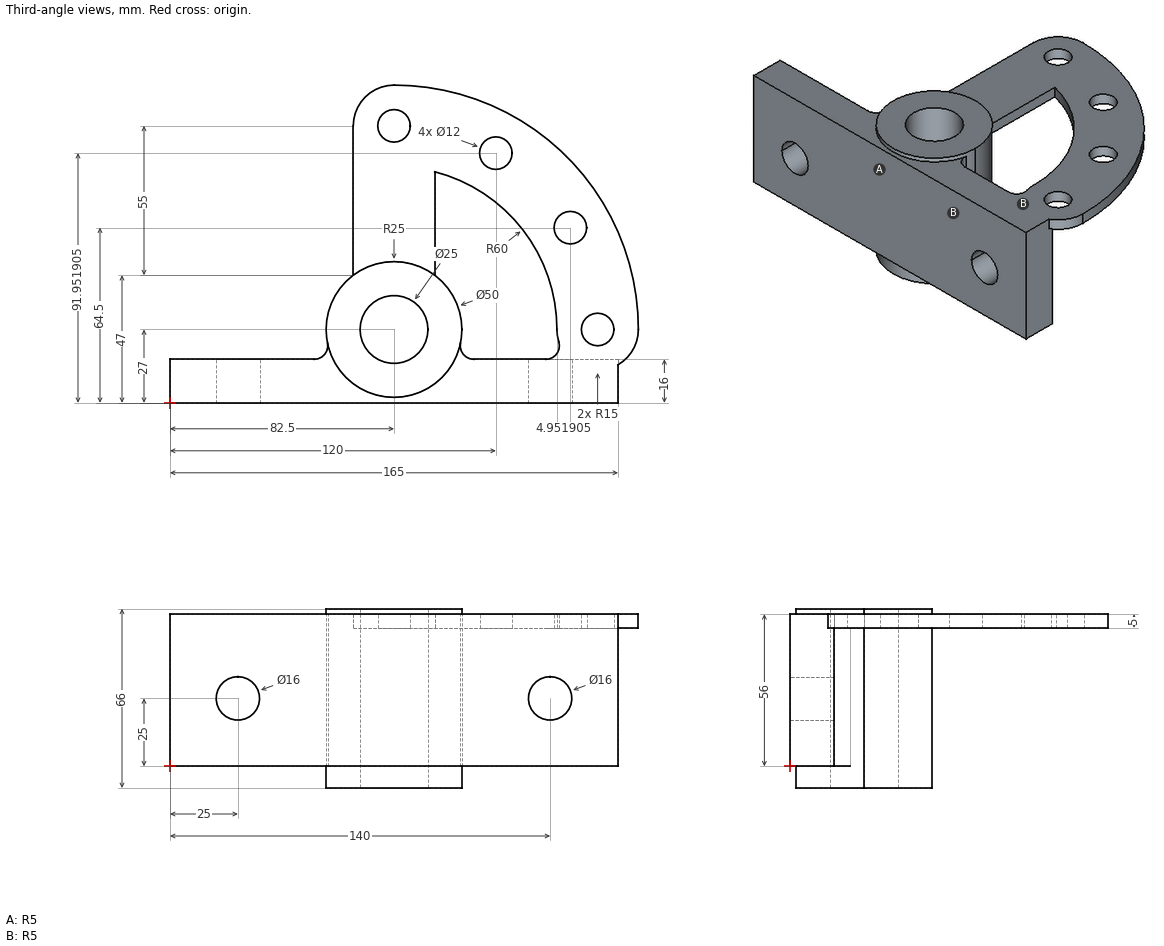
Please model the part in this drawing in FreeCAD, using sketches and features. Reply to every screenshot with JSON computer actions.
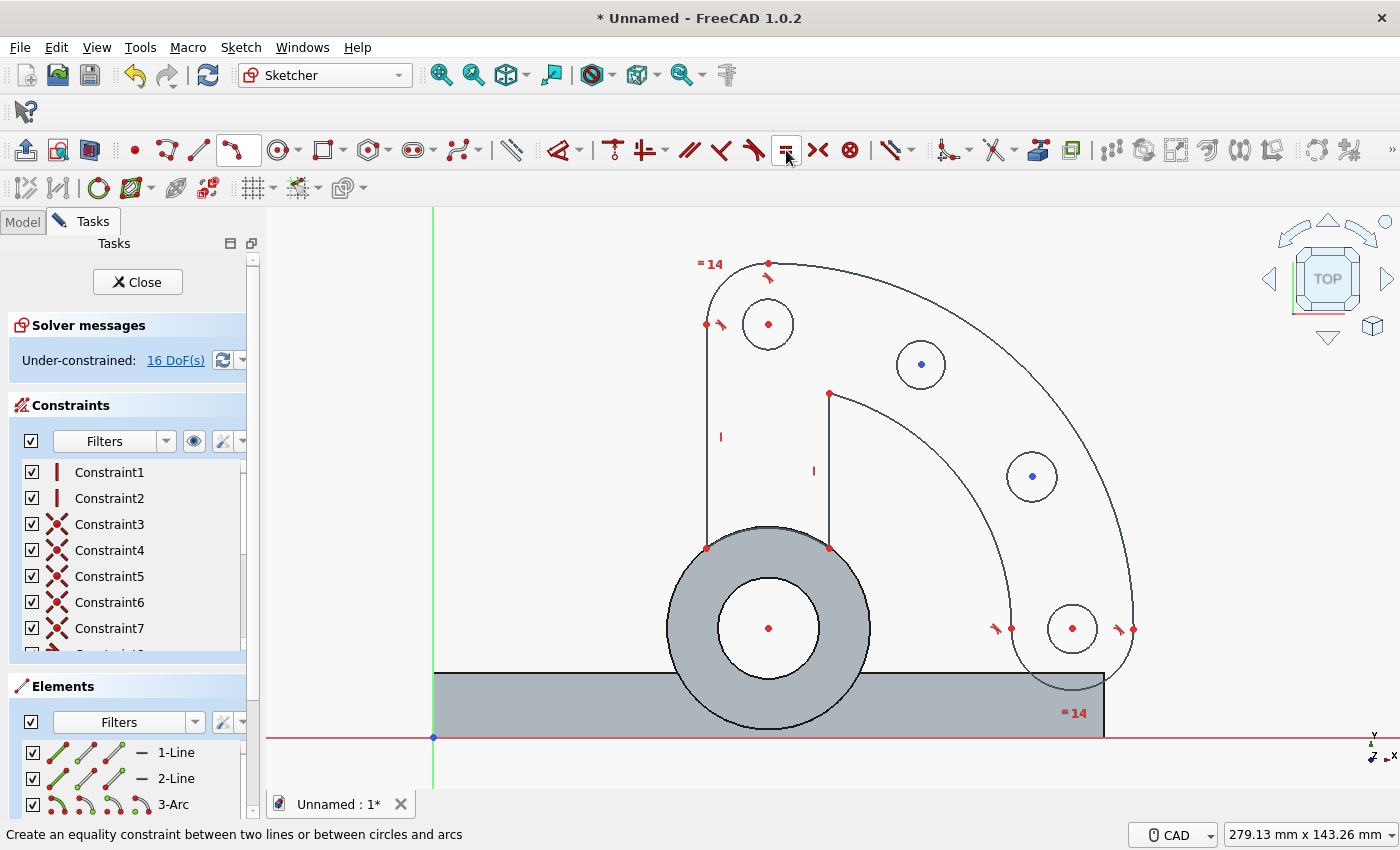
{"action": "left_click", "coordinate": [938, 348]}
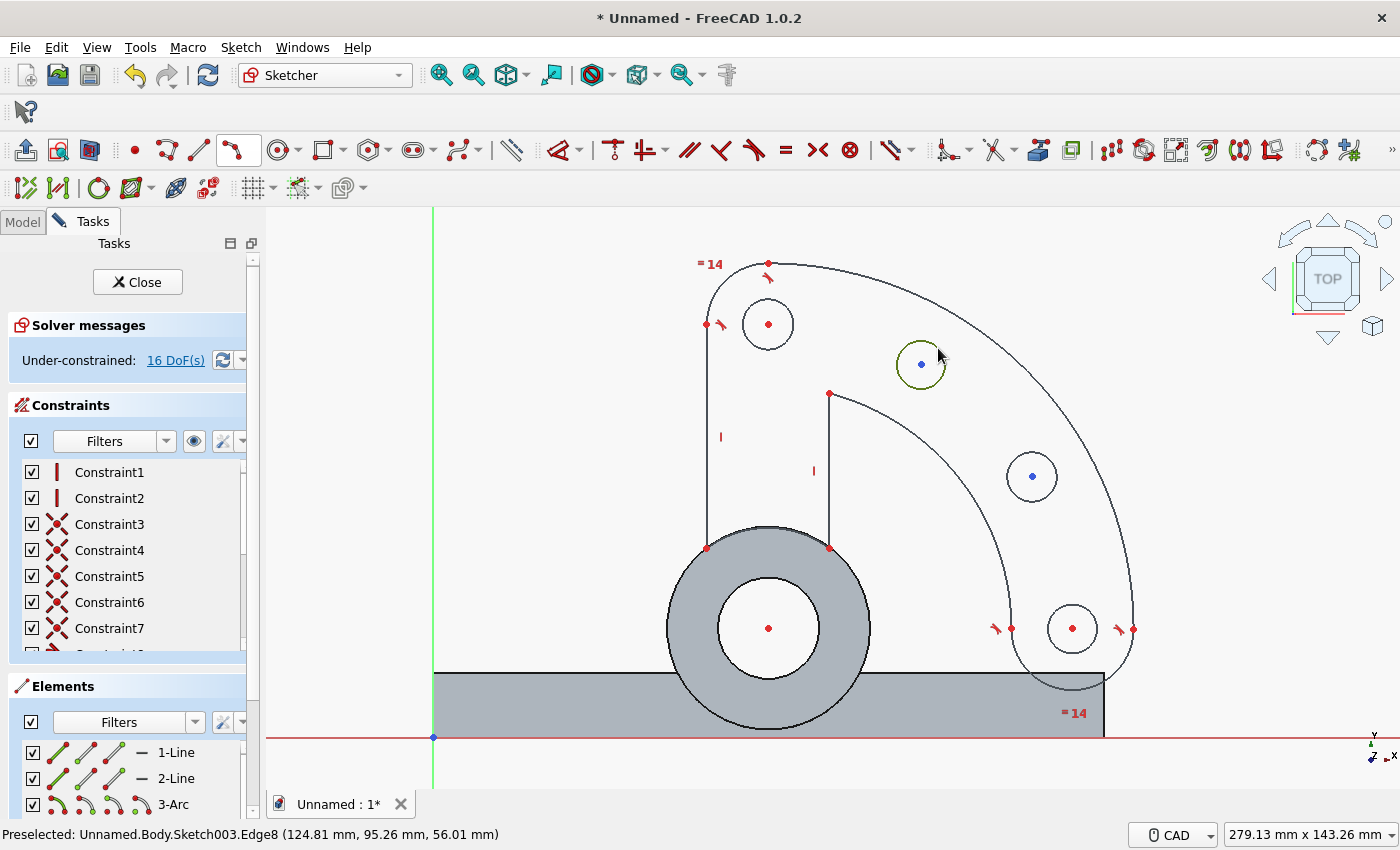
{"action": "left_click", "coordinate": [786, 307]}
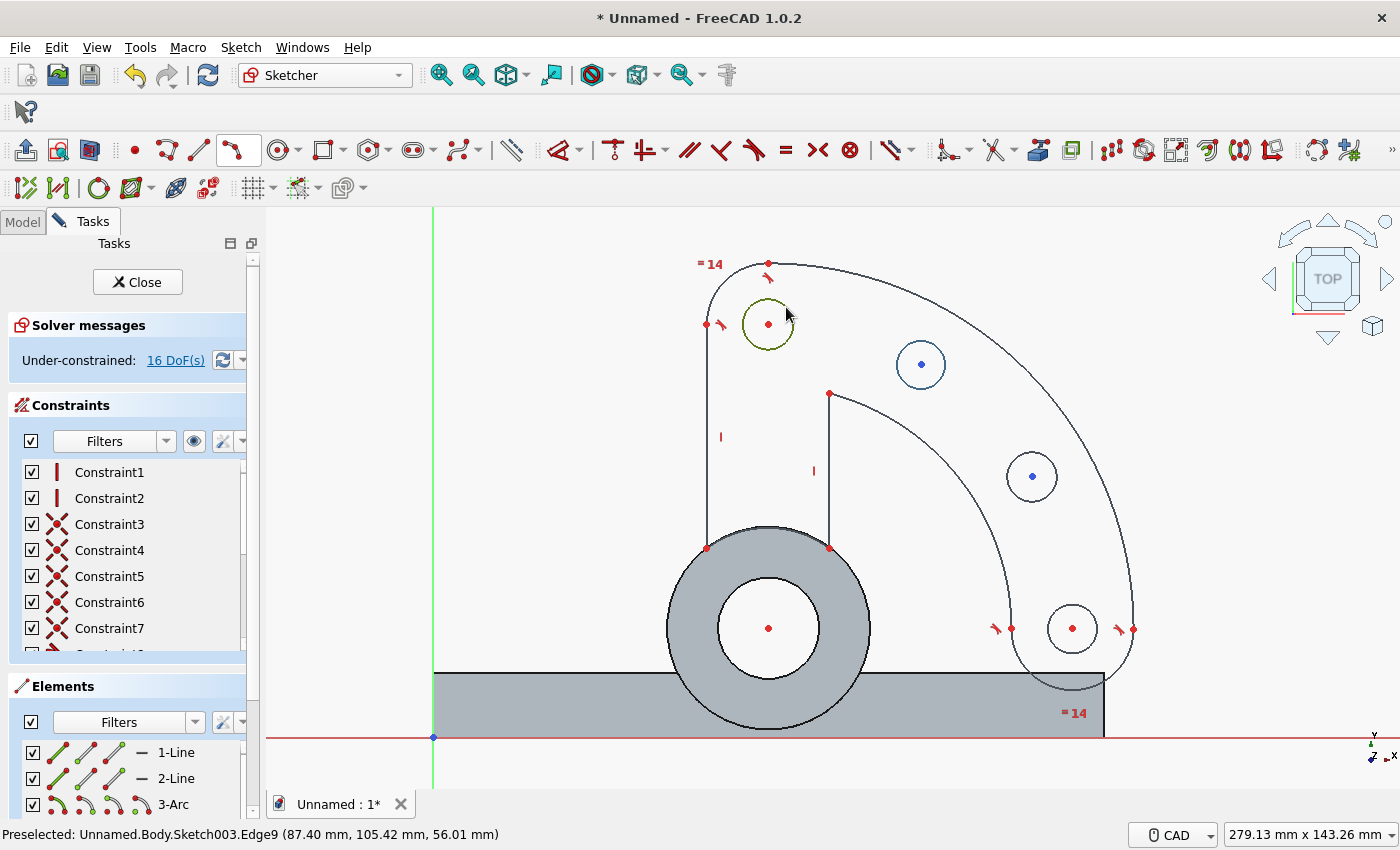
{"action": "left_click", "coordinate": [1090, 612]}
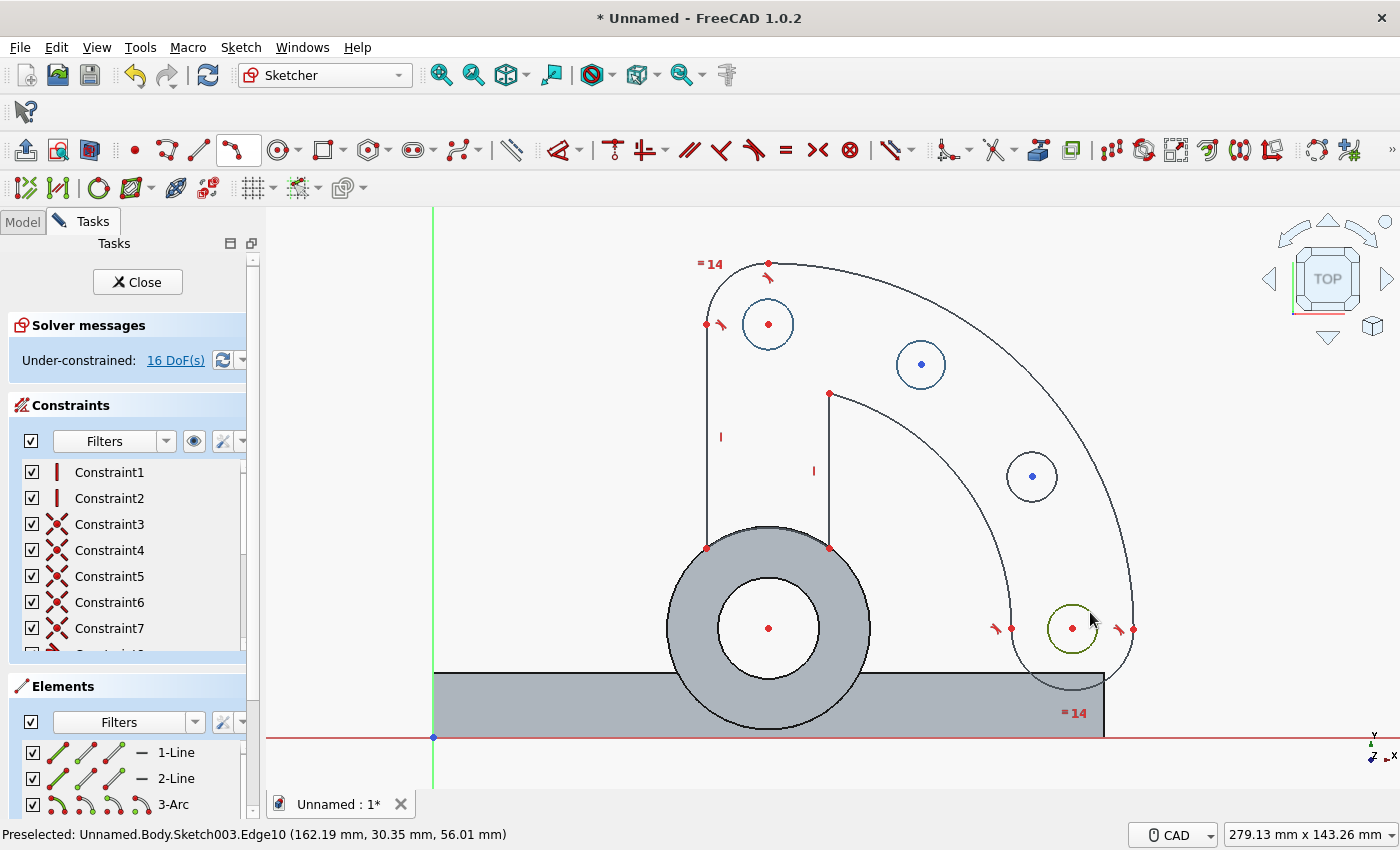
{"action": "left_click", "coordinate": [1049, 459]}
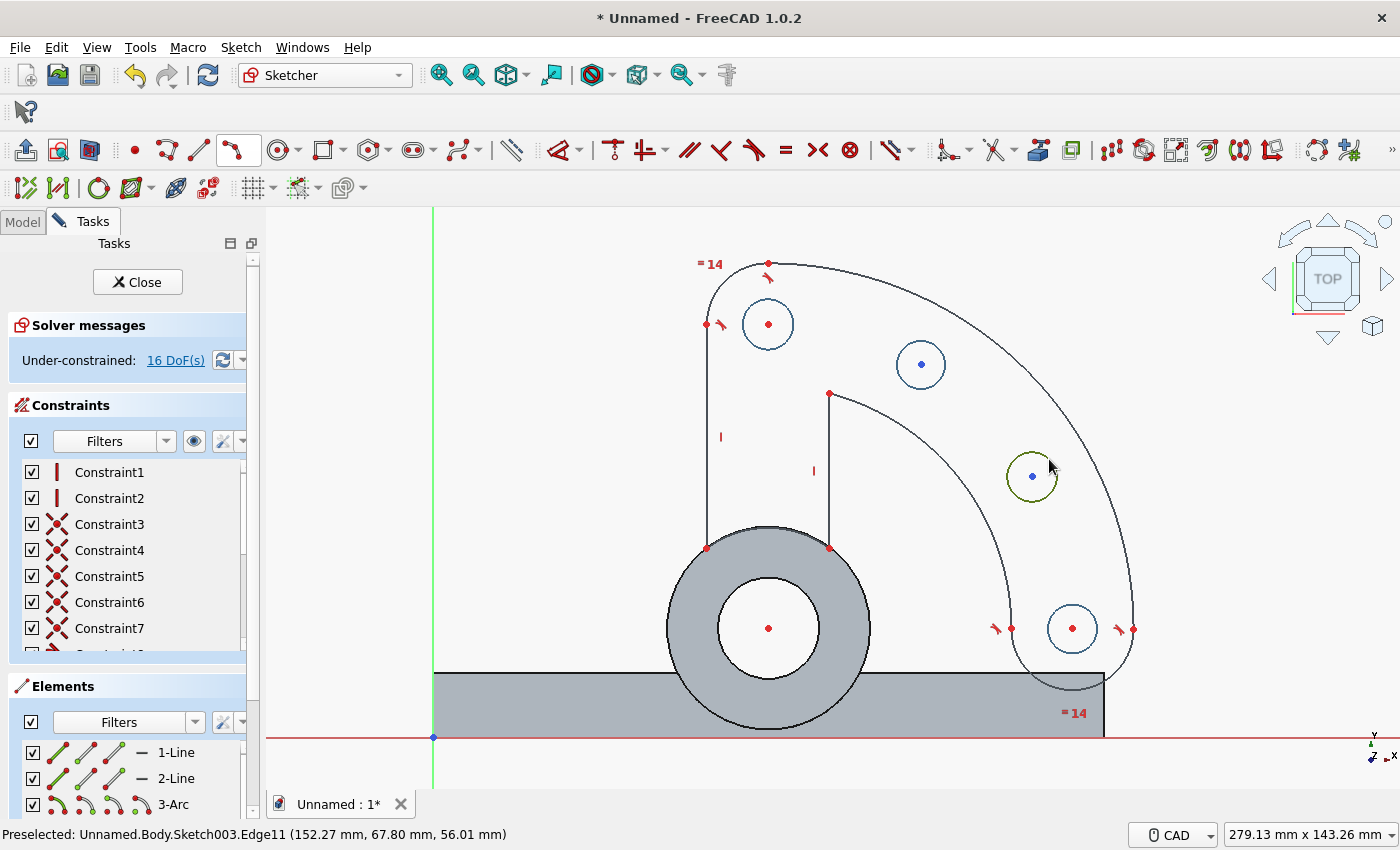
{"action": "key", "text": "e"}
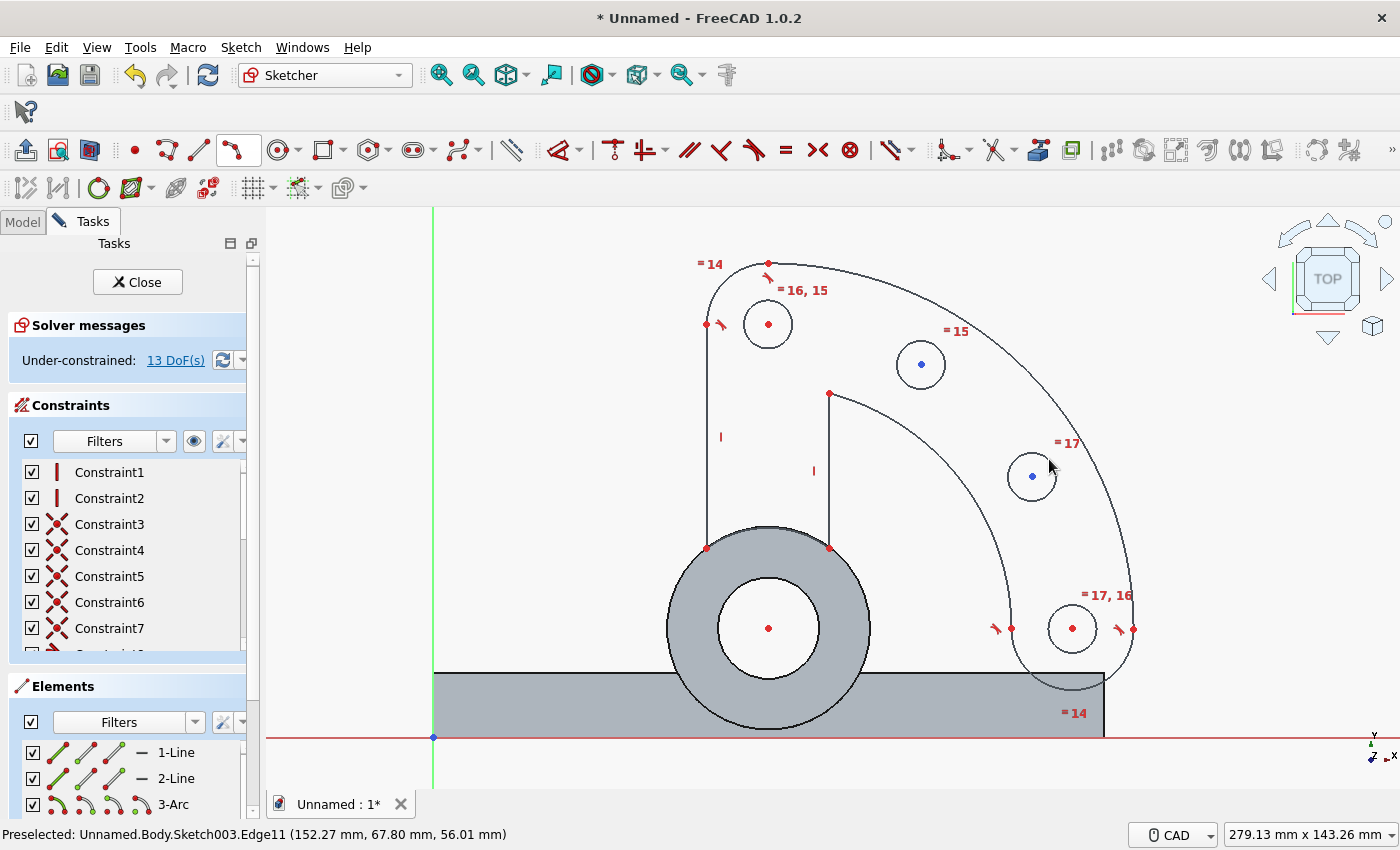
{"action": "key", "text": "d"}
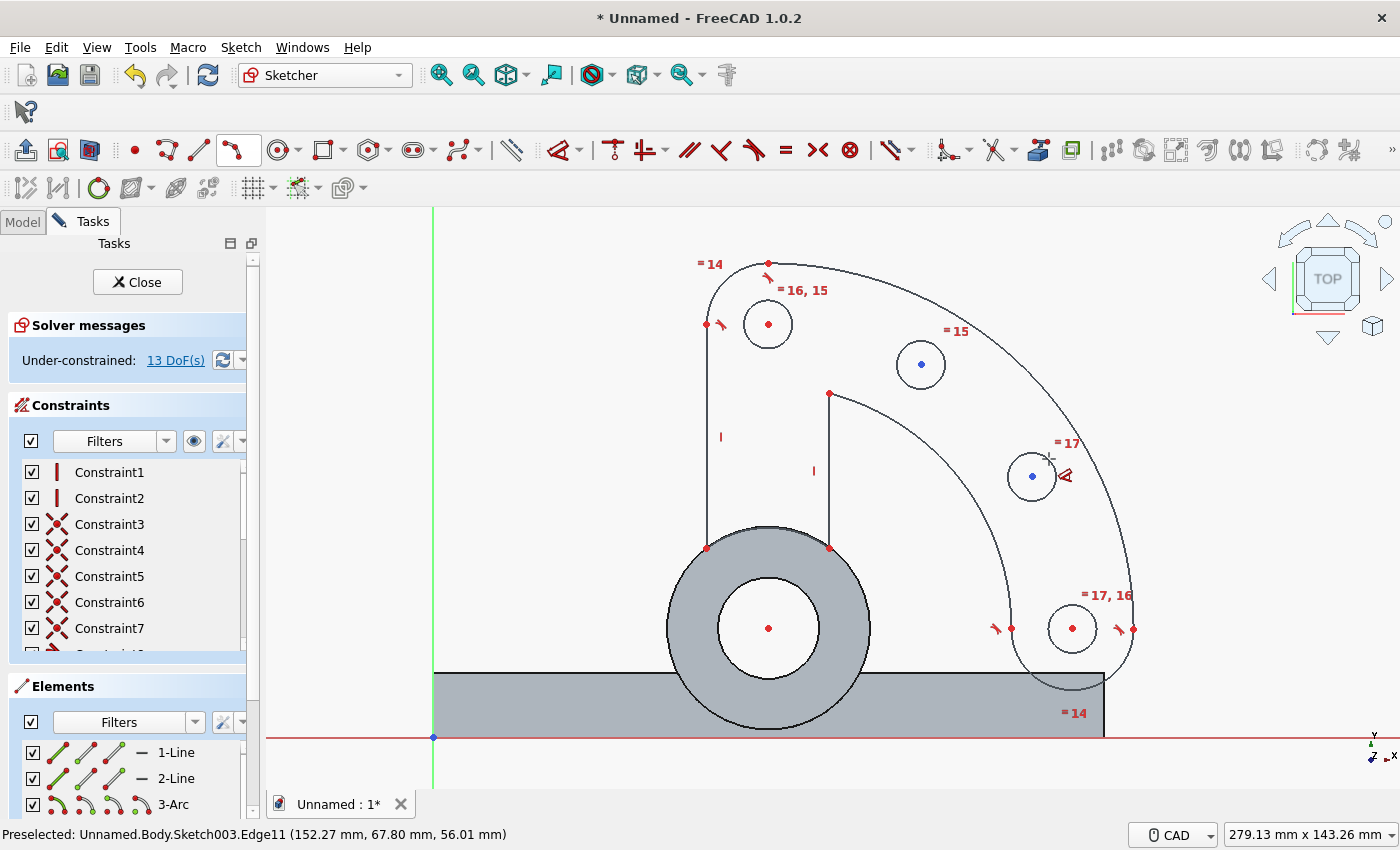
{"action": "left_click", "coordinate": [794, 531]}
{"action": "left_click", "coordinate": [802, 500]}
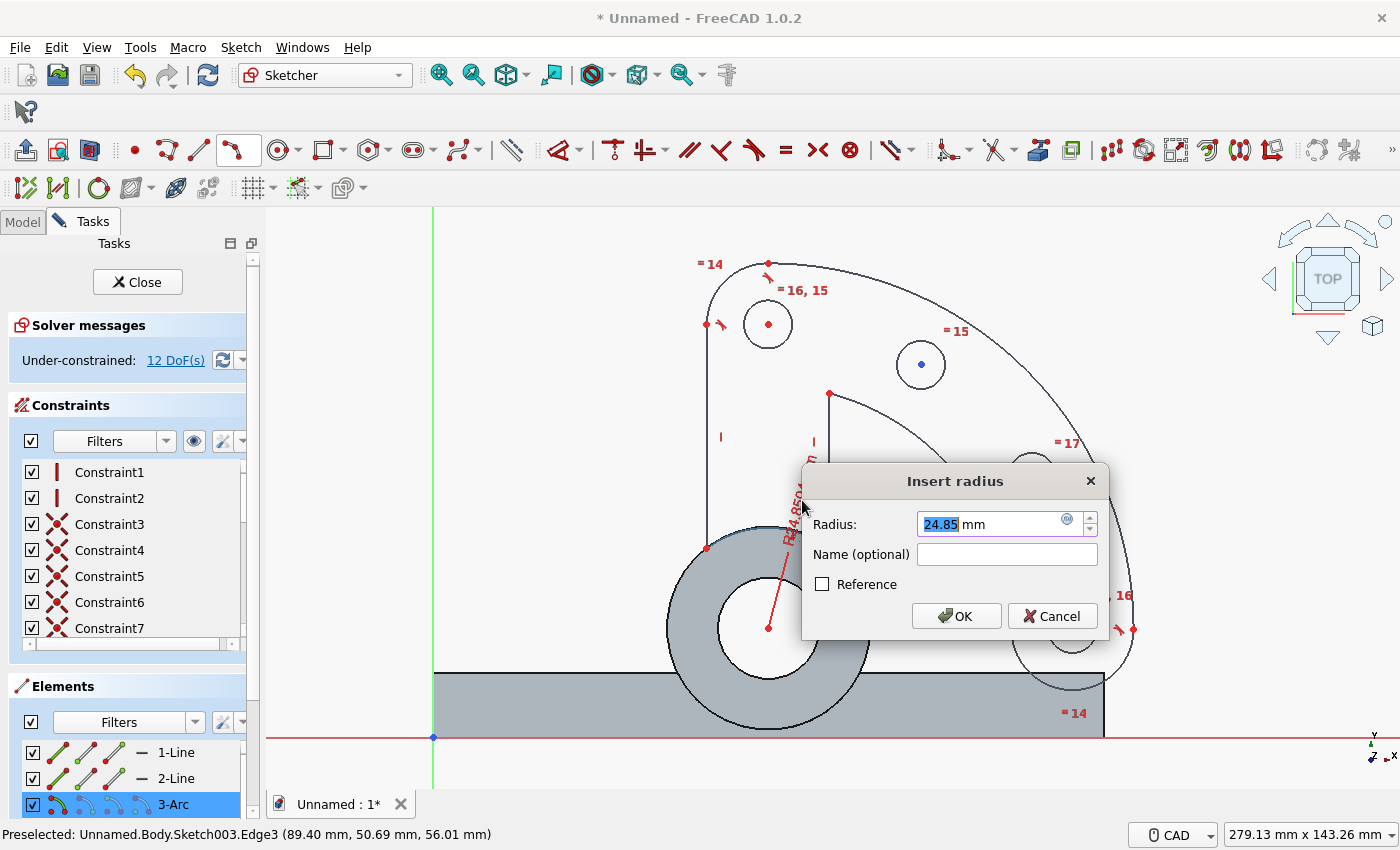
{"action": "type", "text": "25"}
{"action": "key", "text": "Return"}